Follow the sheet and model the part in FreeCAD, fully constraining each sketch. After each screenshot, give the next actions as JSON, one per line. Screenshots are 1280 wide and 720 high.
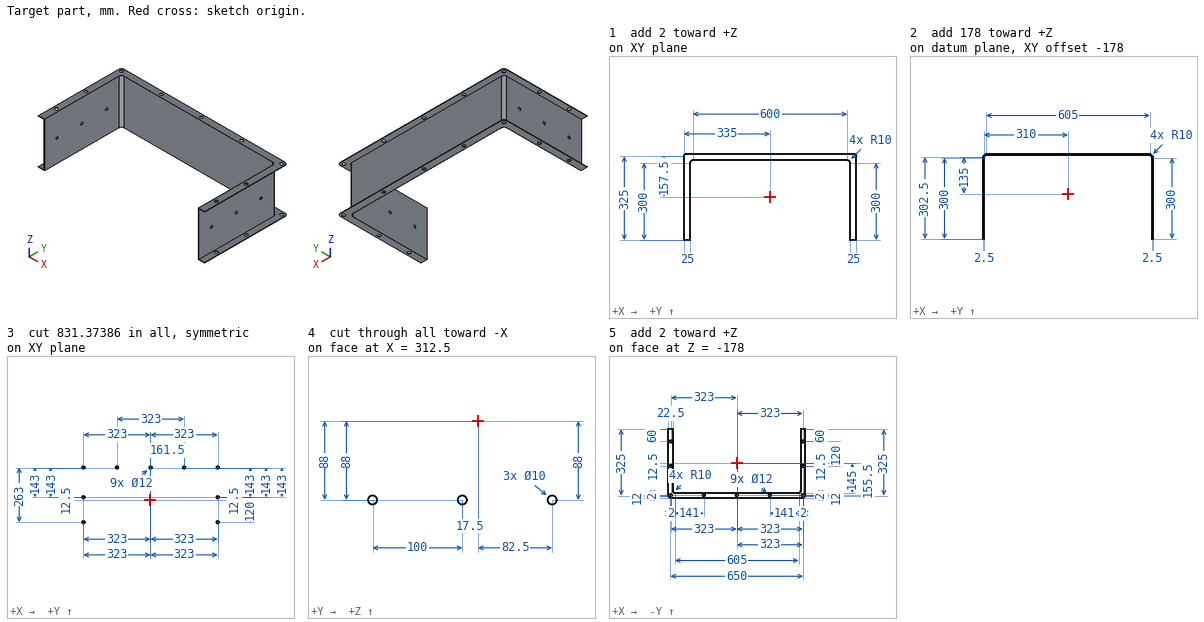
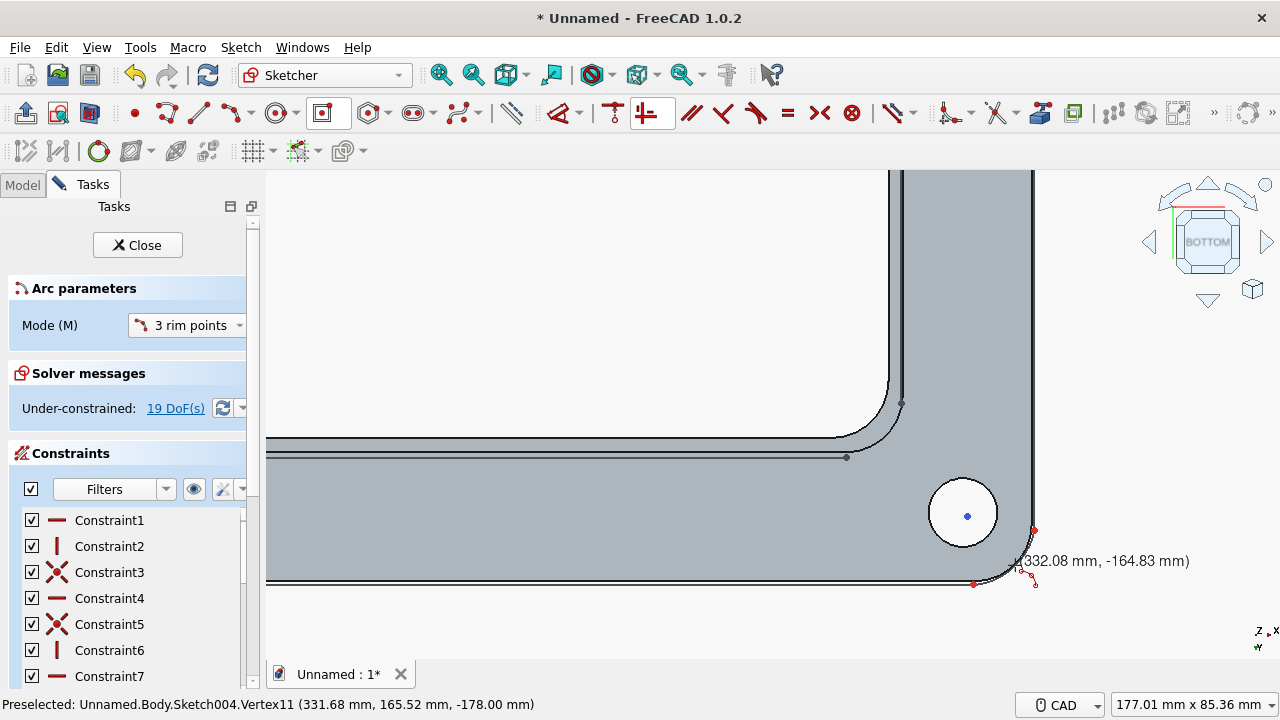
{"action": "scroll", "coordinate": [1020, 571], "scroll_direction": "down", "scroll_amount": 9}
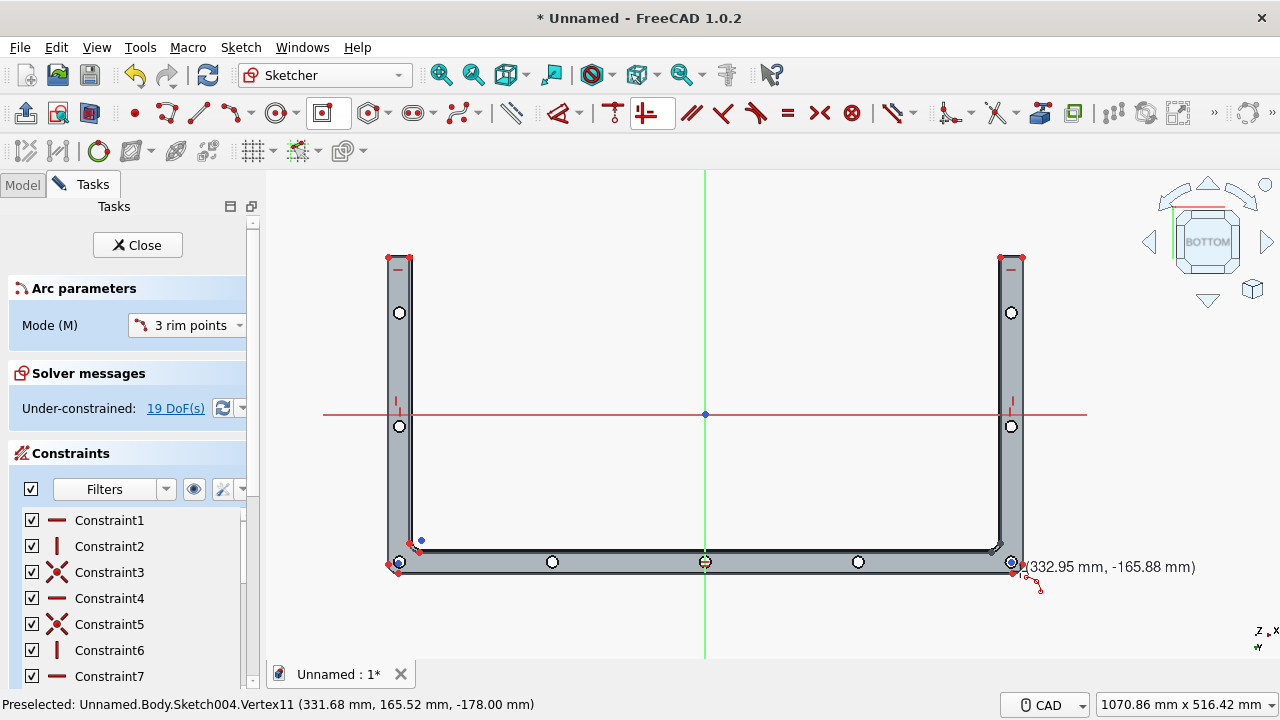
{"action": "left_click", "coordinate": [1001, 544]}
{"action": "left_click", "coordinate": [992, 553]}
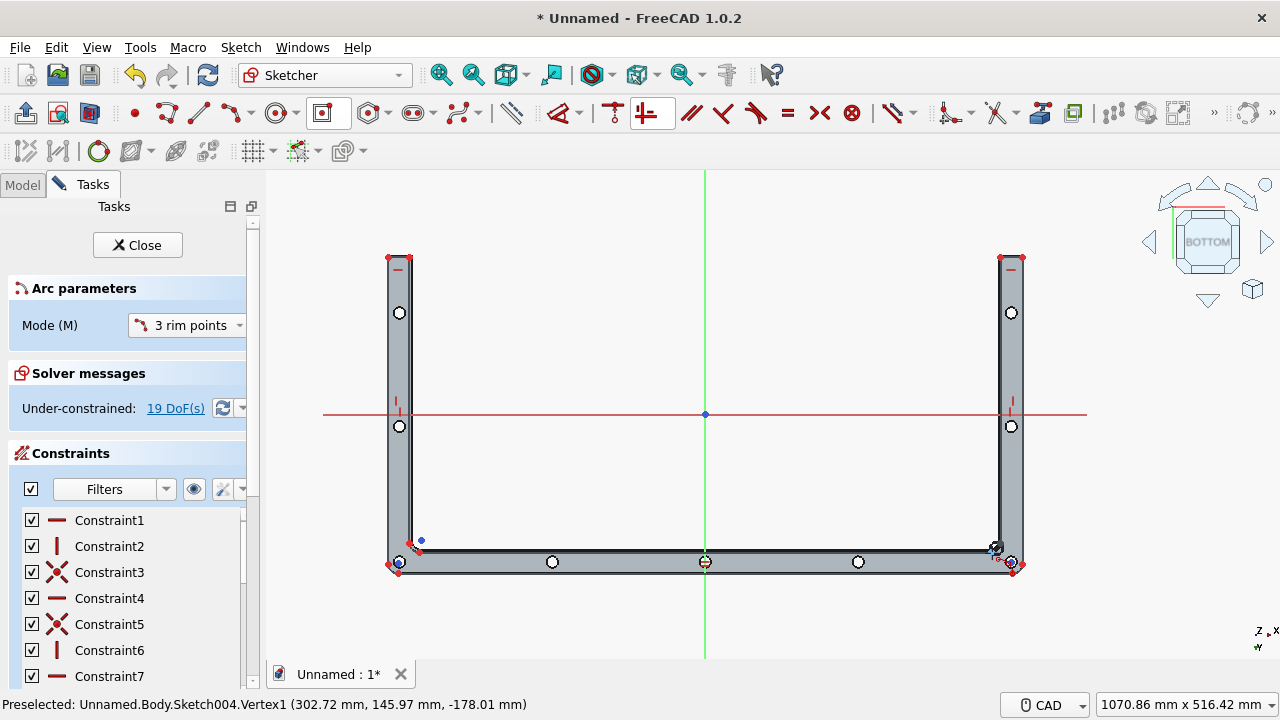
{"action": "scroll", "coordinate": [998, 549], "scroll_direction": "up", "scroll_amount": 9}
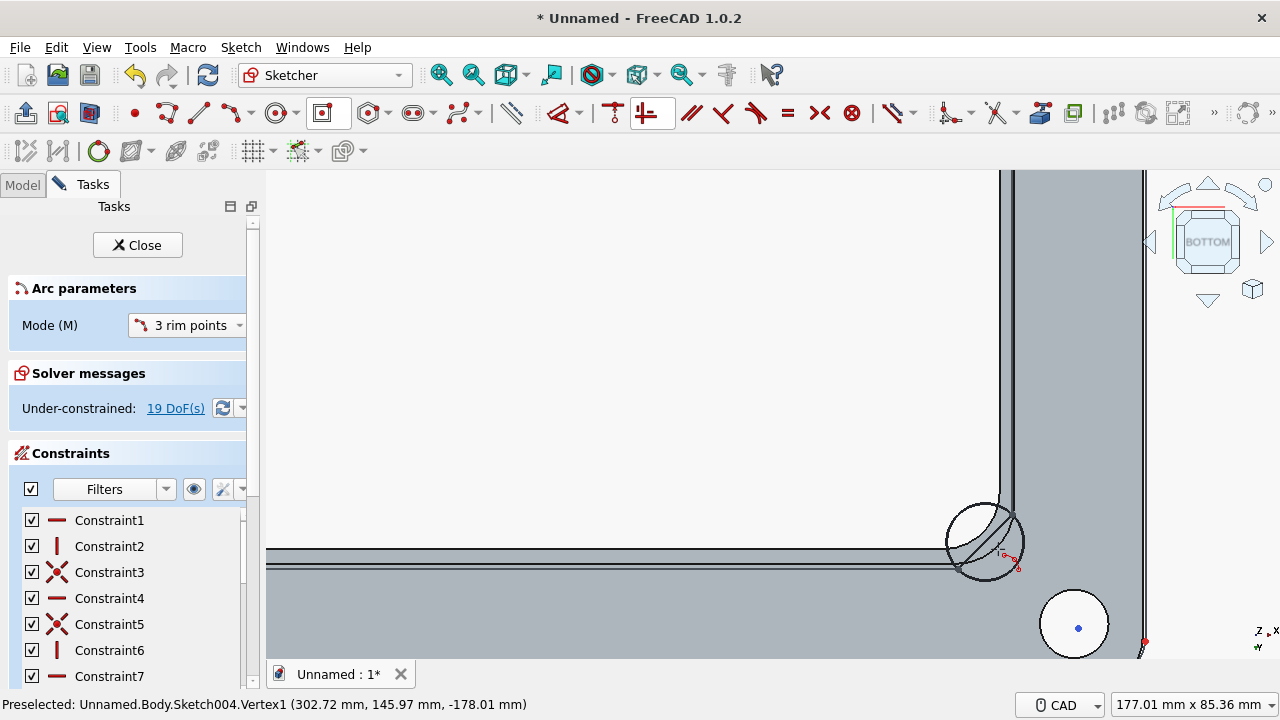
{"action": "left_click", "coordinate": [997, 547]}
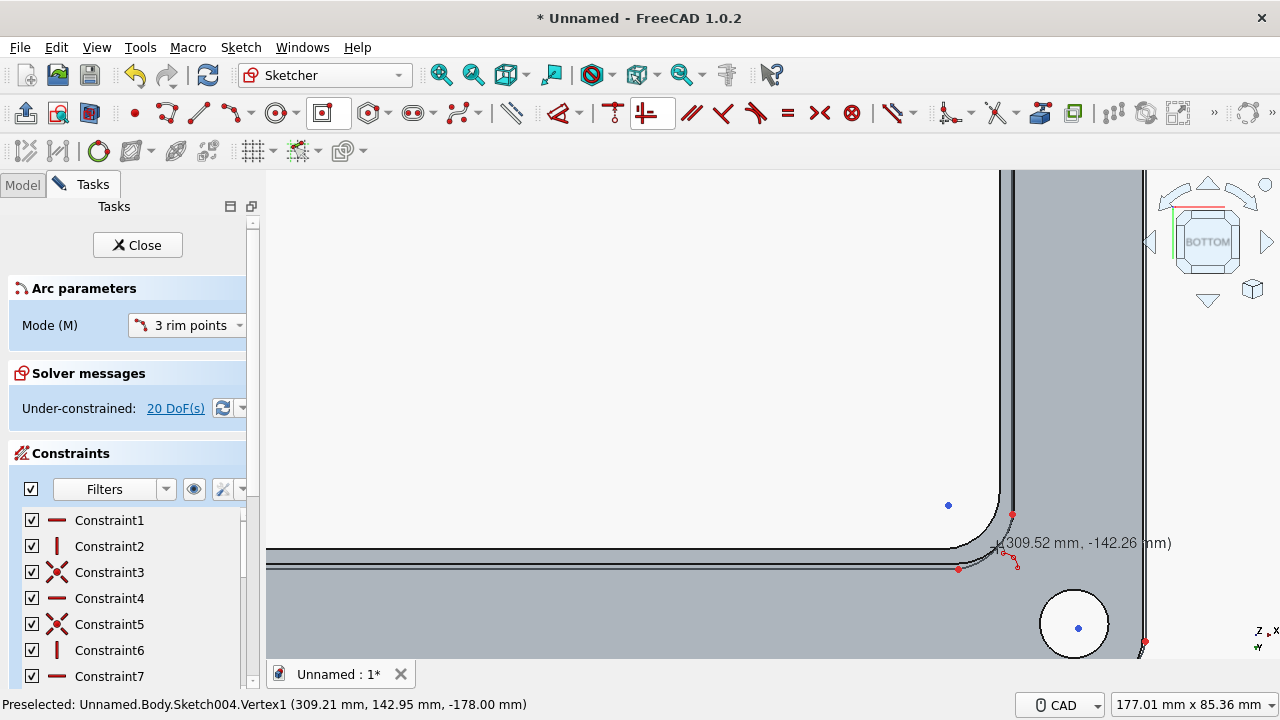
{"action": "left_click", "coordinate": [276, 114]}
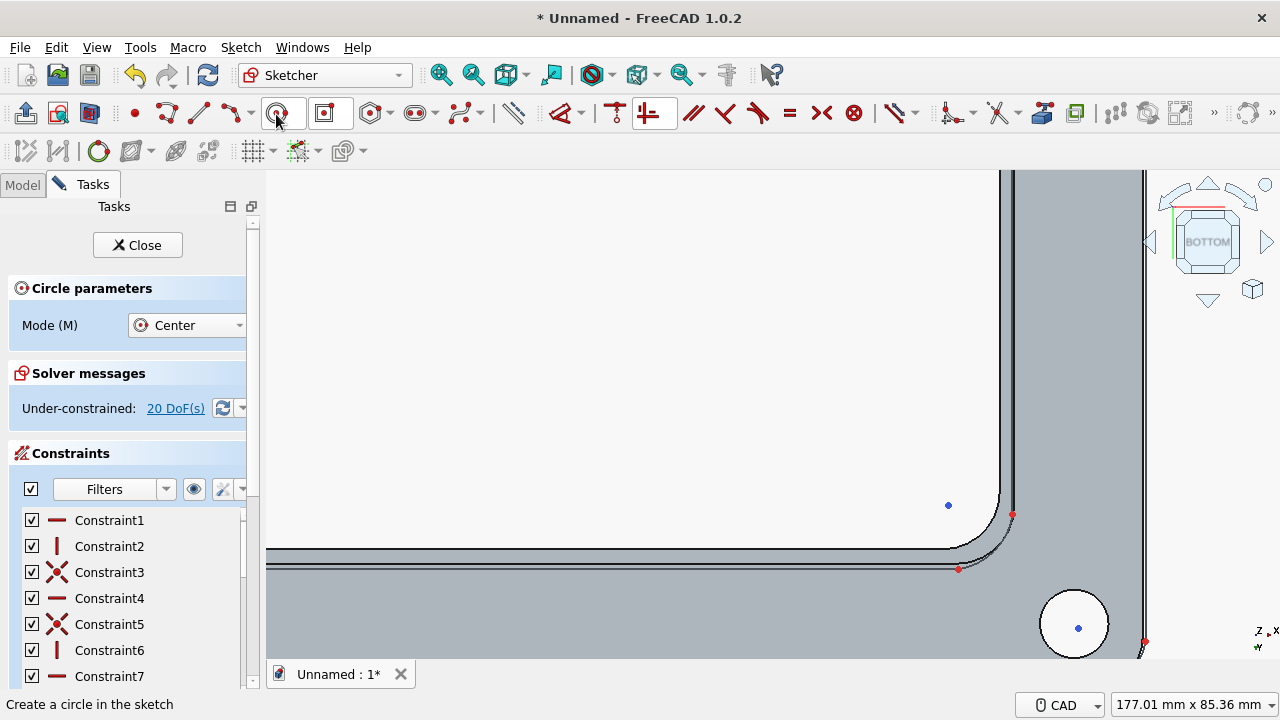
{"action": "scroll", "coordinate": [998, 549], "scroll_direction": "down", "scroll_amount": 9}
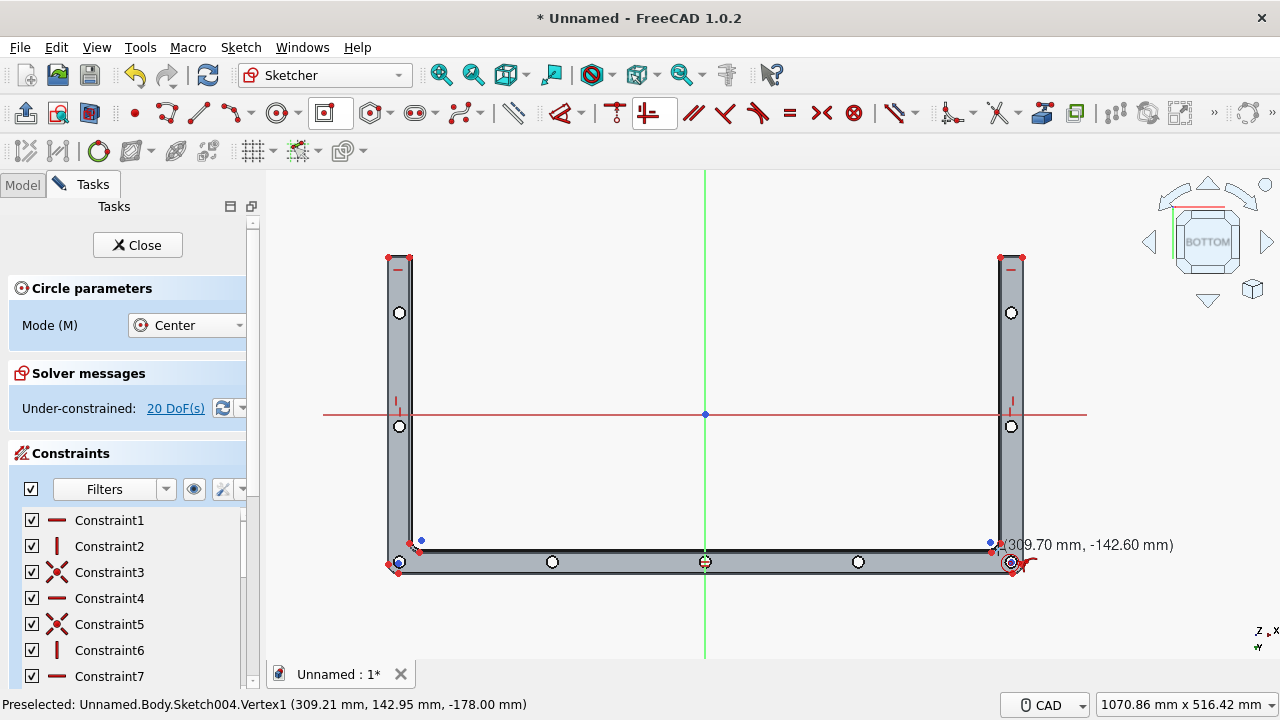
{"action": "scroll", "coordinate": [1011, 313], "scroll_direction": "up", "scroll_amount": 7}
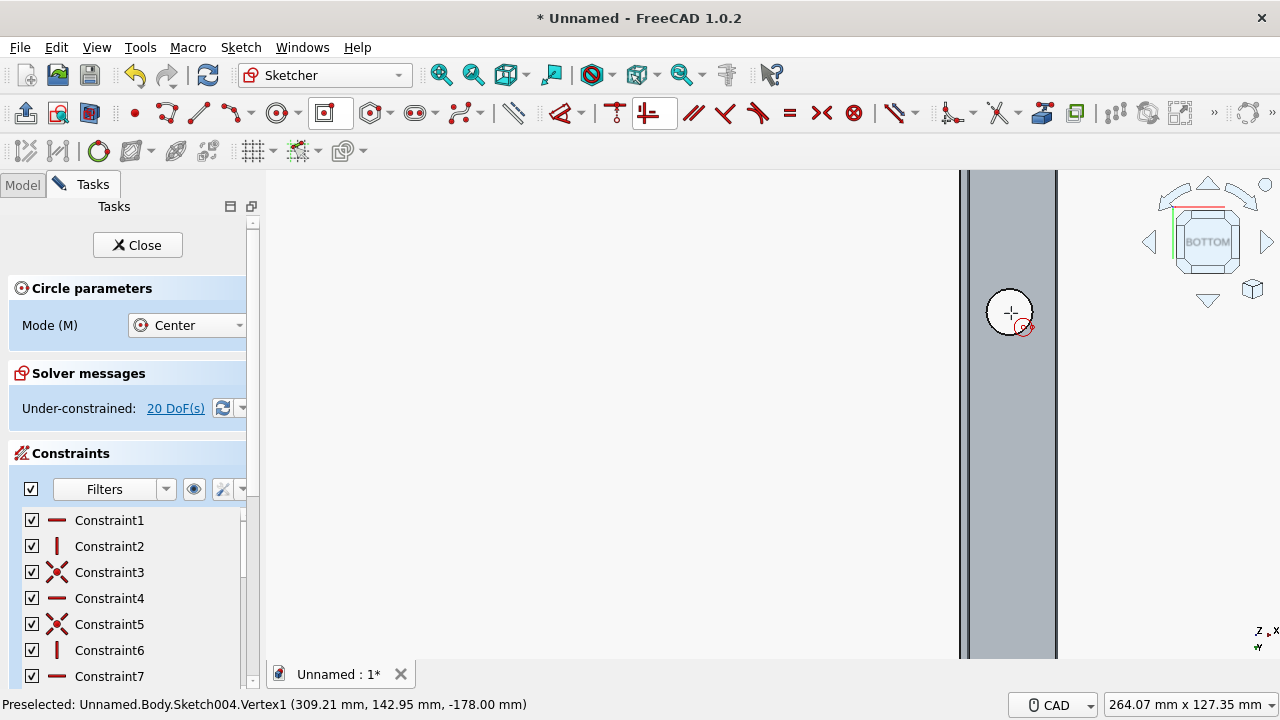
{"action": "left_click", "coordinate": [1010, 312]}
{"action": "mouse_move", "coordinate": [1026, 296]}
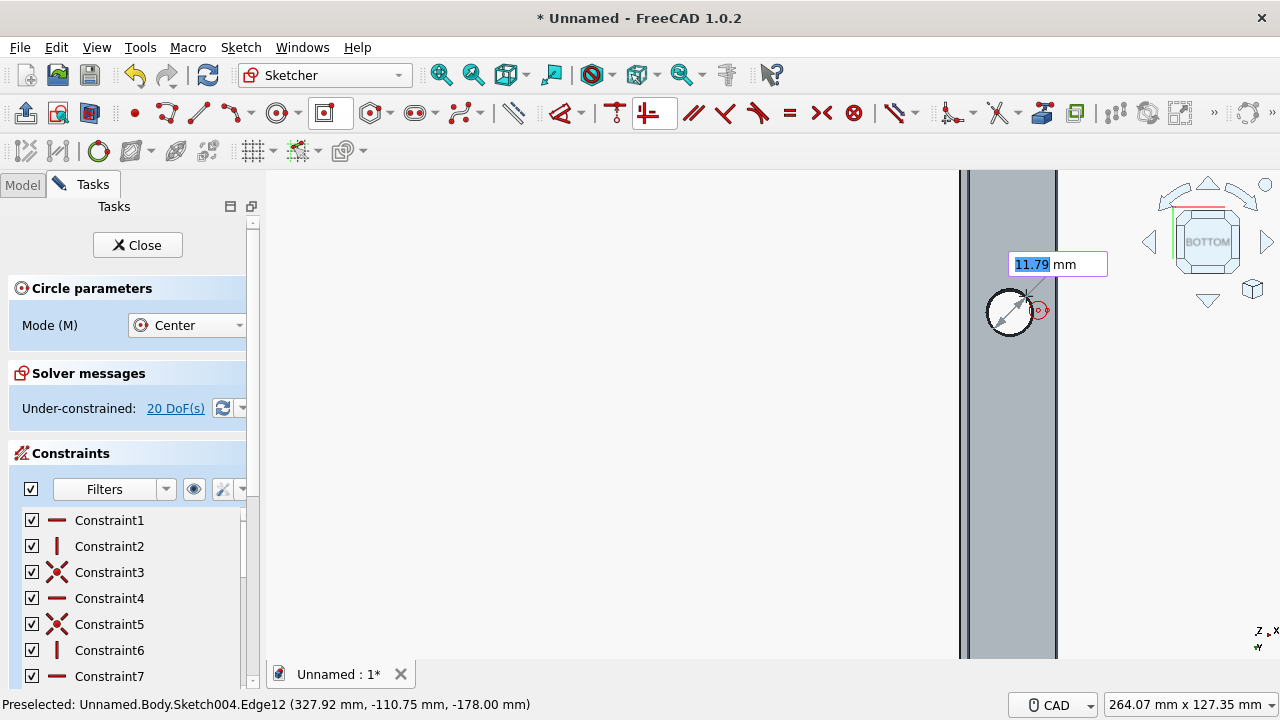
{"action": "type", "text": "12"}
{"action": "key", "text": "Return"}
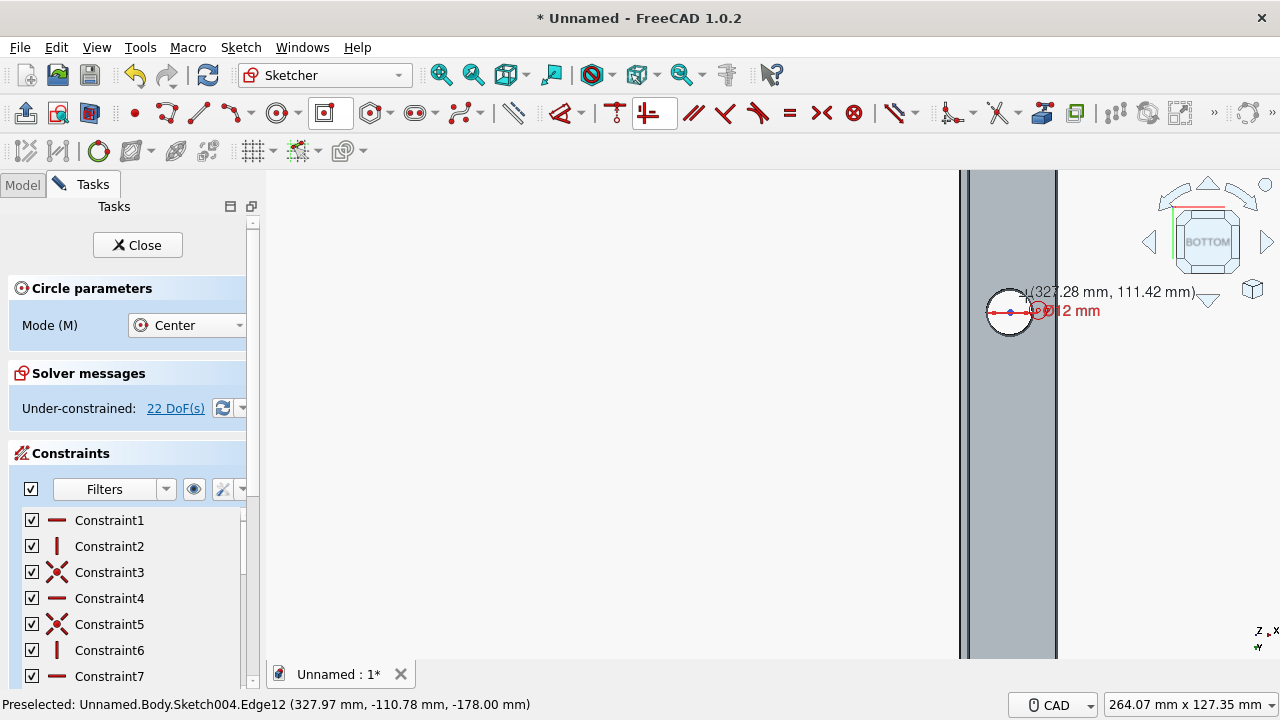
{"action": "scroll", "coordinate": [1011, 313], "scroll_direction": "down", "scroll_amount": 7}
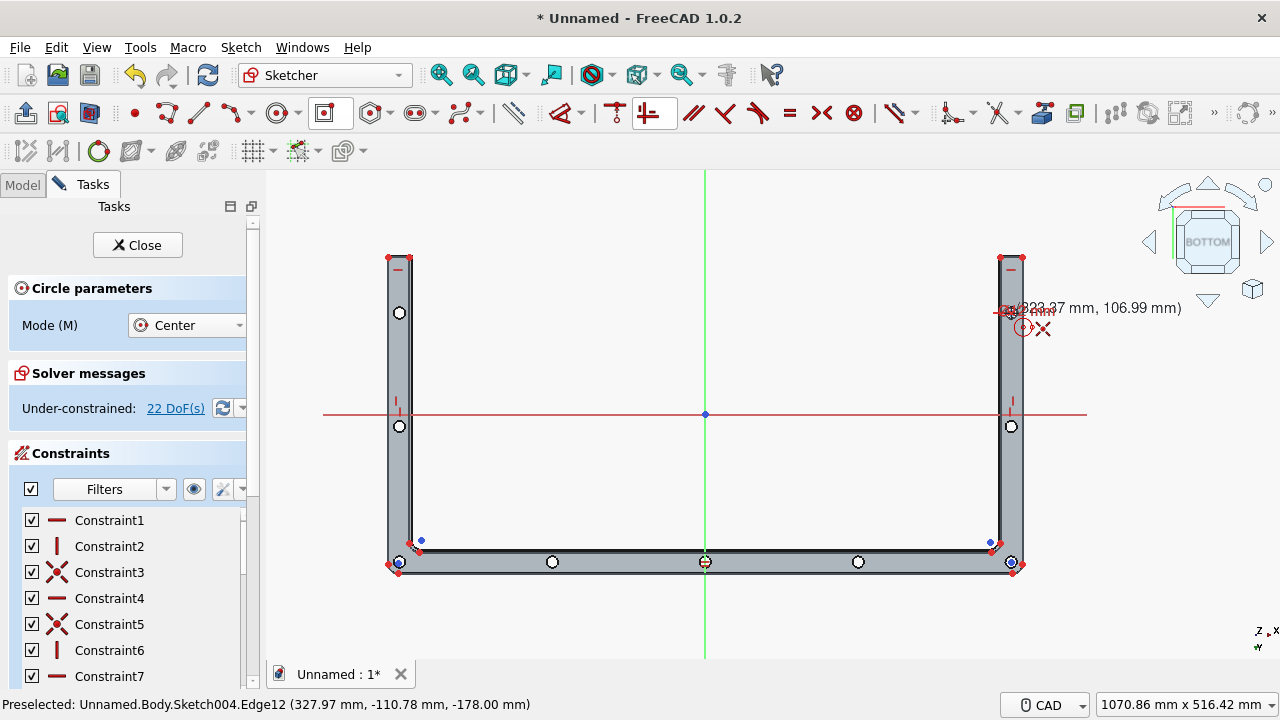
{"action": "scroll", "coordinate": [1011, 427], "scroll_direction": "up", "scroll_amount": 7}